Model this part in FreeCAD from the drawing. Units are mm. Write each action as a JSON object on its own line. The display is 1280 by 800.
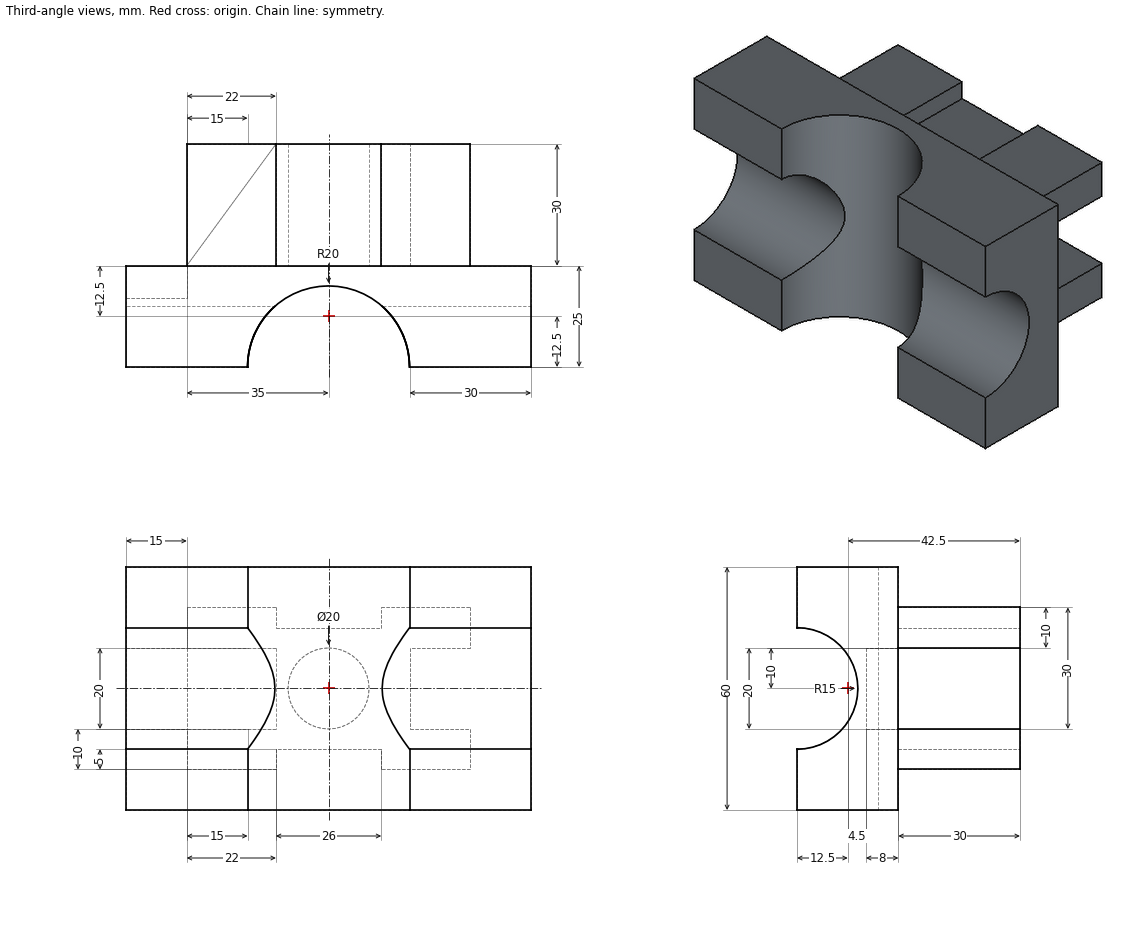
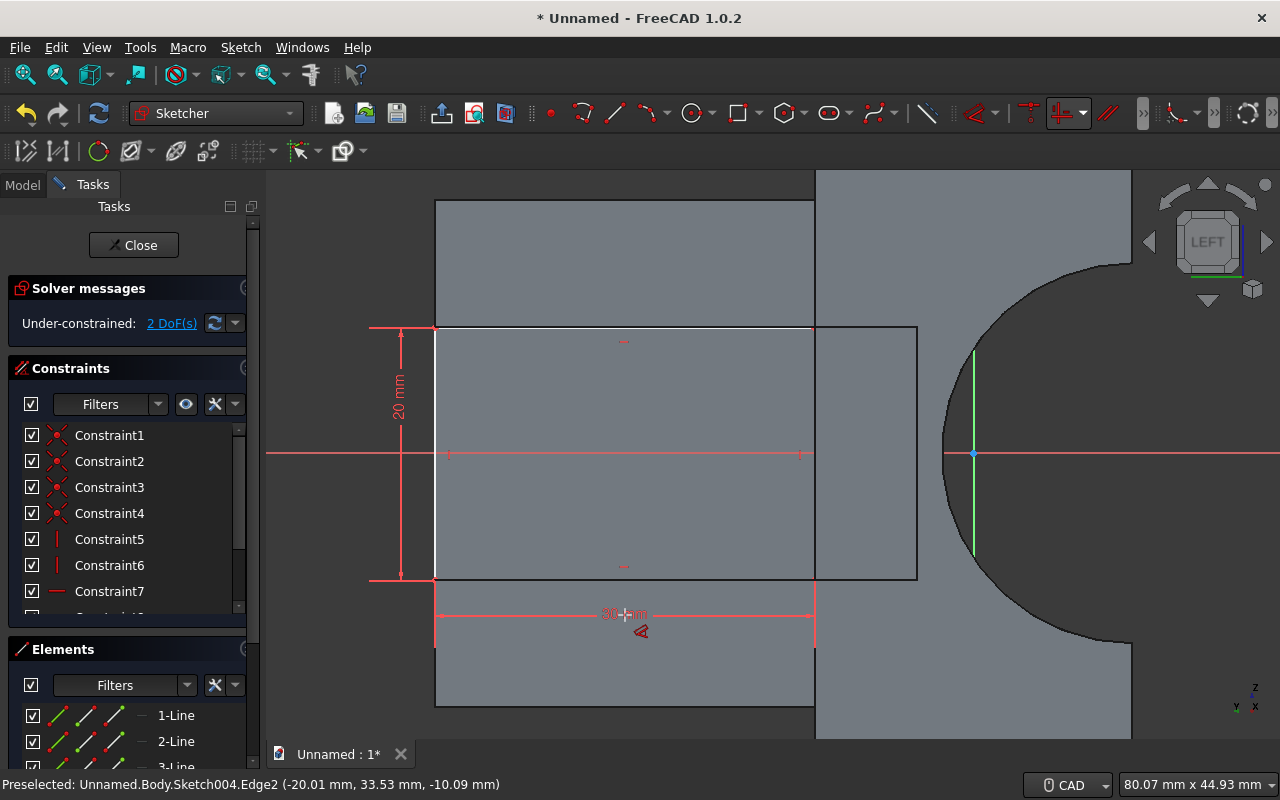
{"action": "left_click", "coordinate": [435, 328]}
{"action": "left_click", "coordinate": [401, 362]}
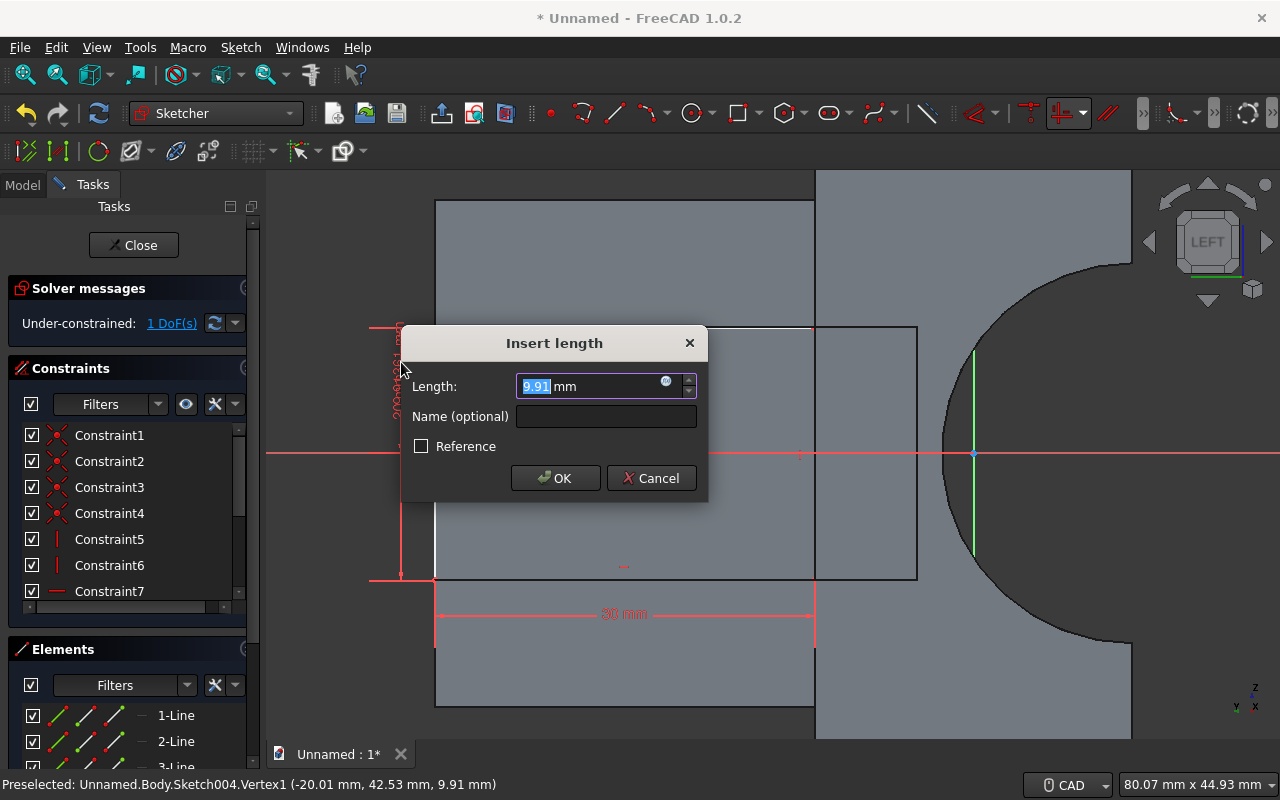
{"action": "type", "text": "10"}
{"action": "key", "text": "Return"}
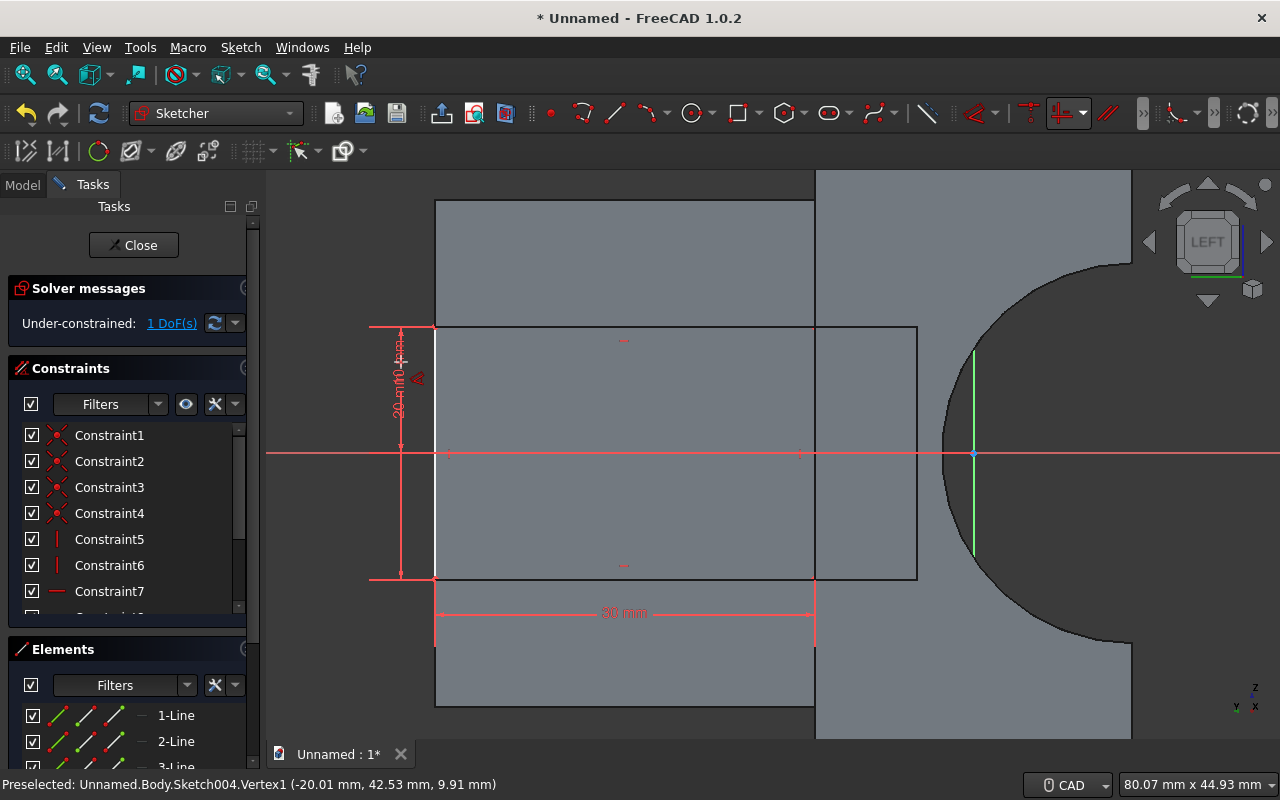
{"action": "left_click", "coordinate": [435, 327]}
{"action": "left_click", "coordinate": [704, 293]}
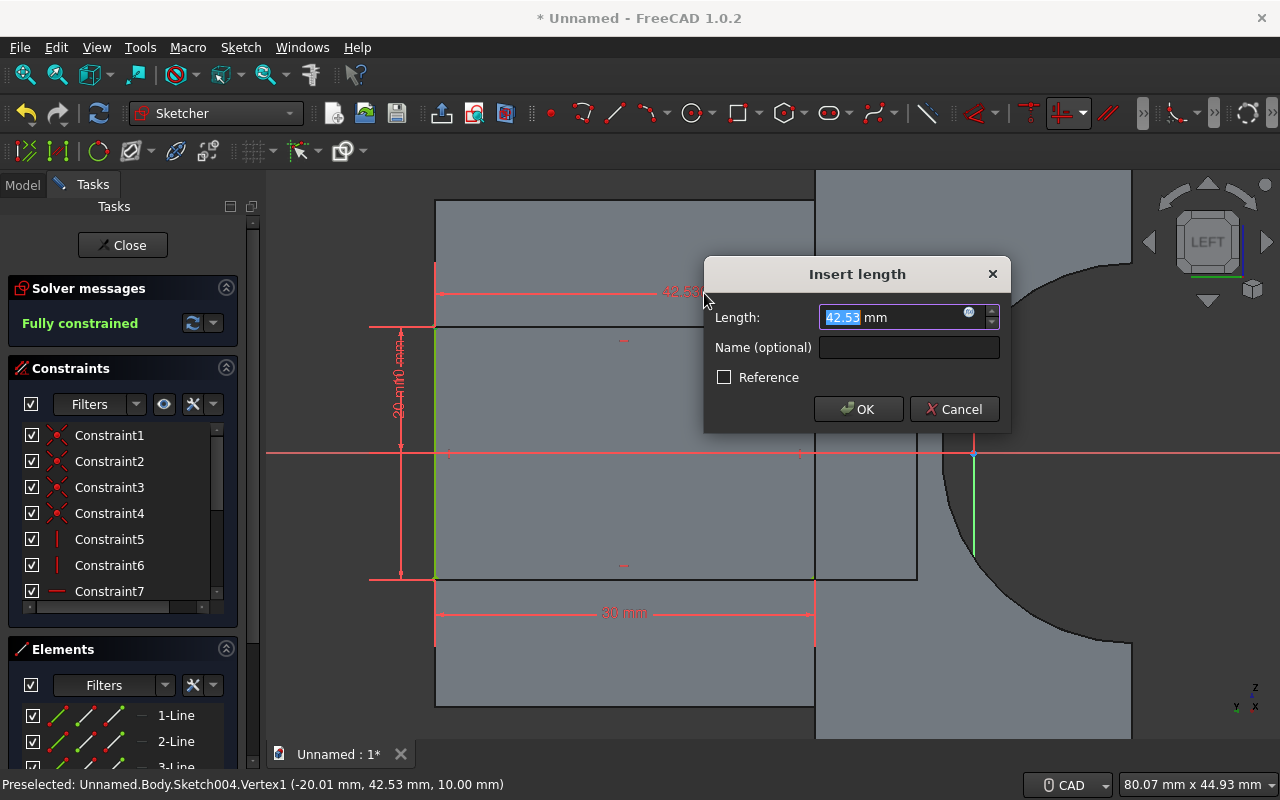
{"action": "type", "text": "42.5"}
{"action": "key", "text": "Return"}
{"action": "key", "text": "Escape"}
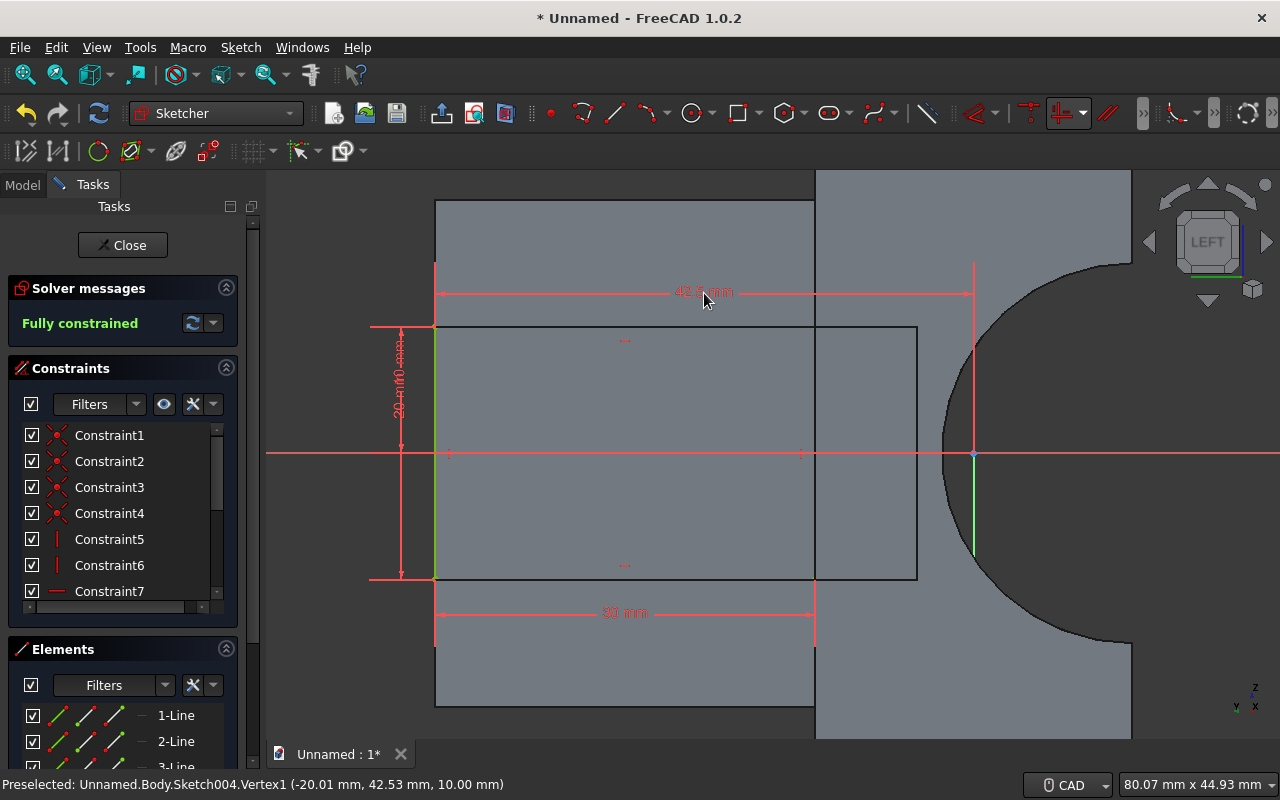
{"action": "left_click", "coordinate": [123, 245]}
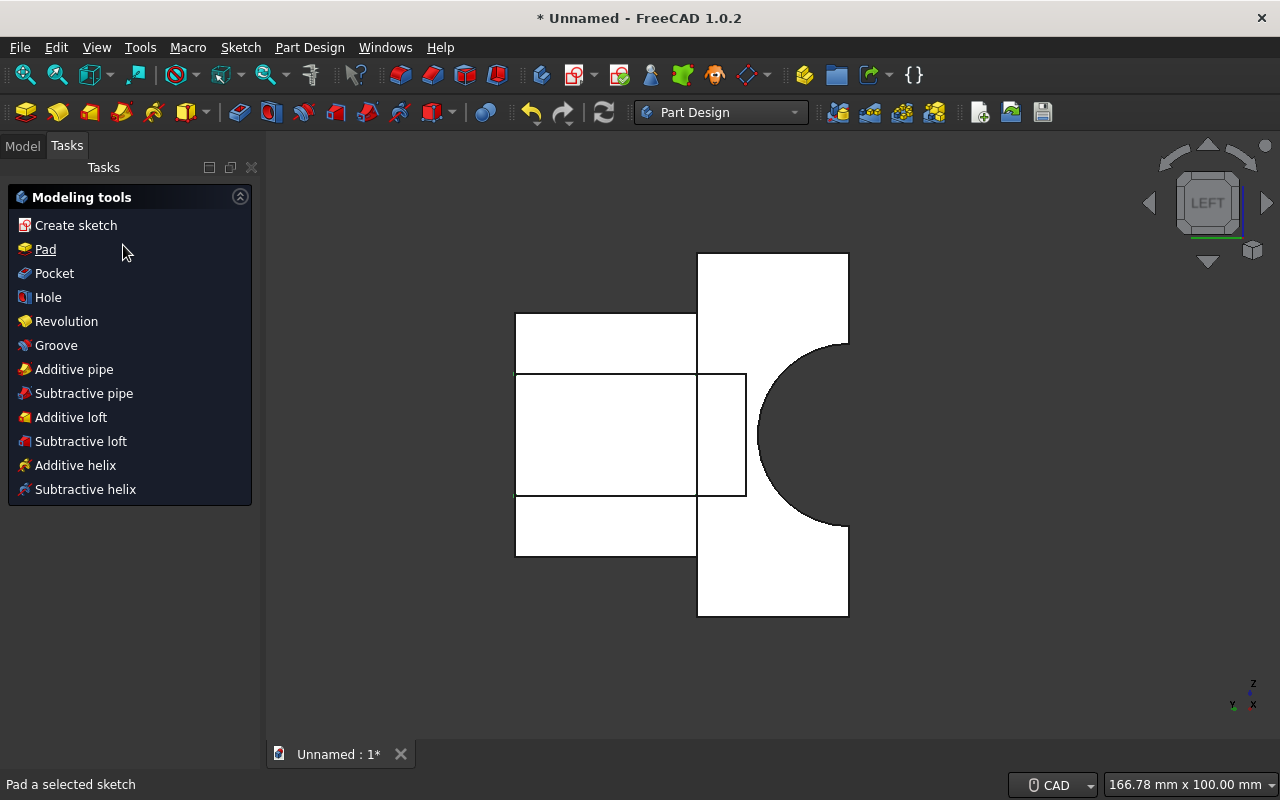
{"action": "left_click", "coordinate": [26, 112]}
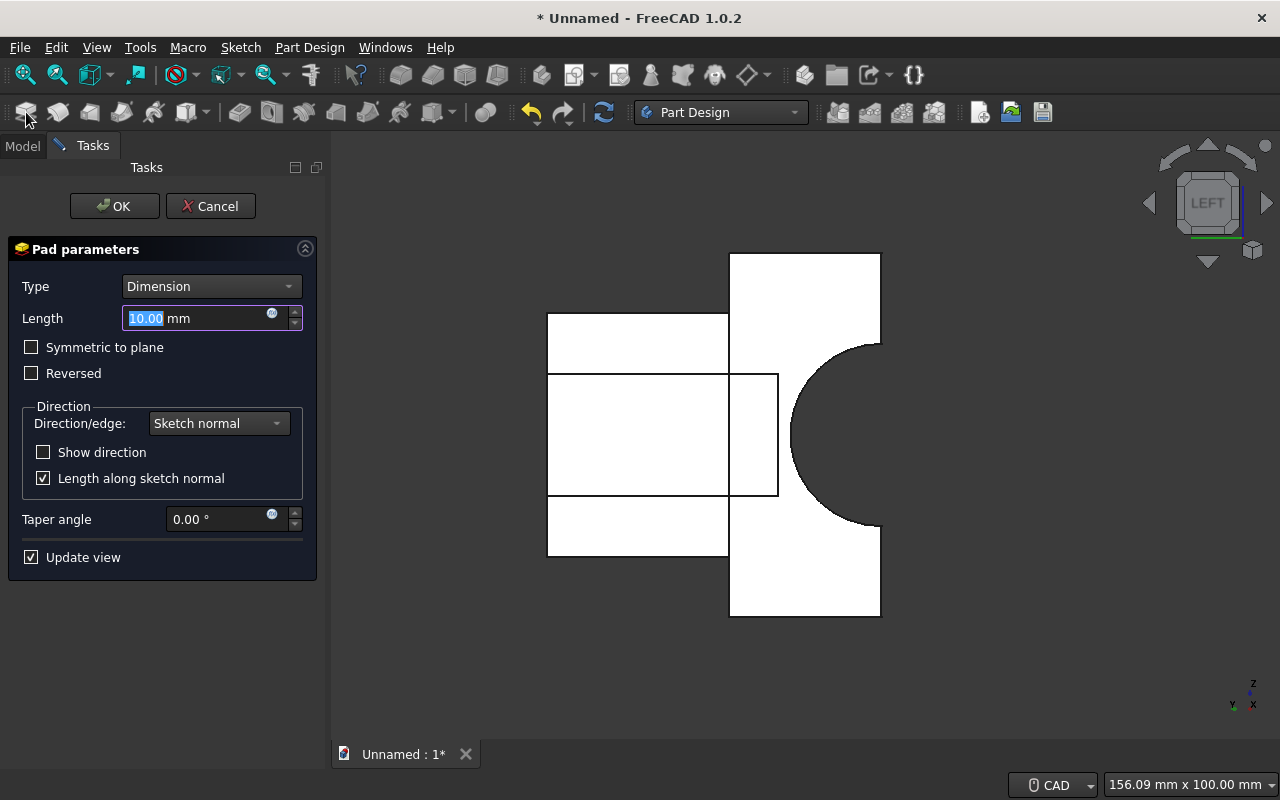
{"action": "type", "text": "15"}
{"action": "key", "text": "Tab"}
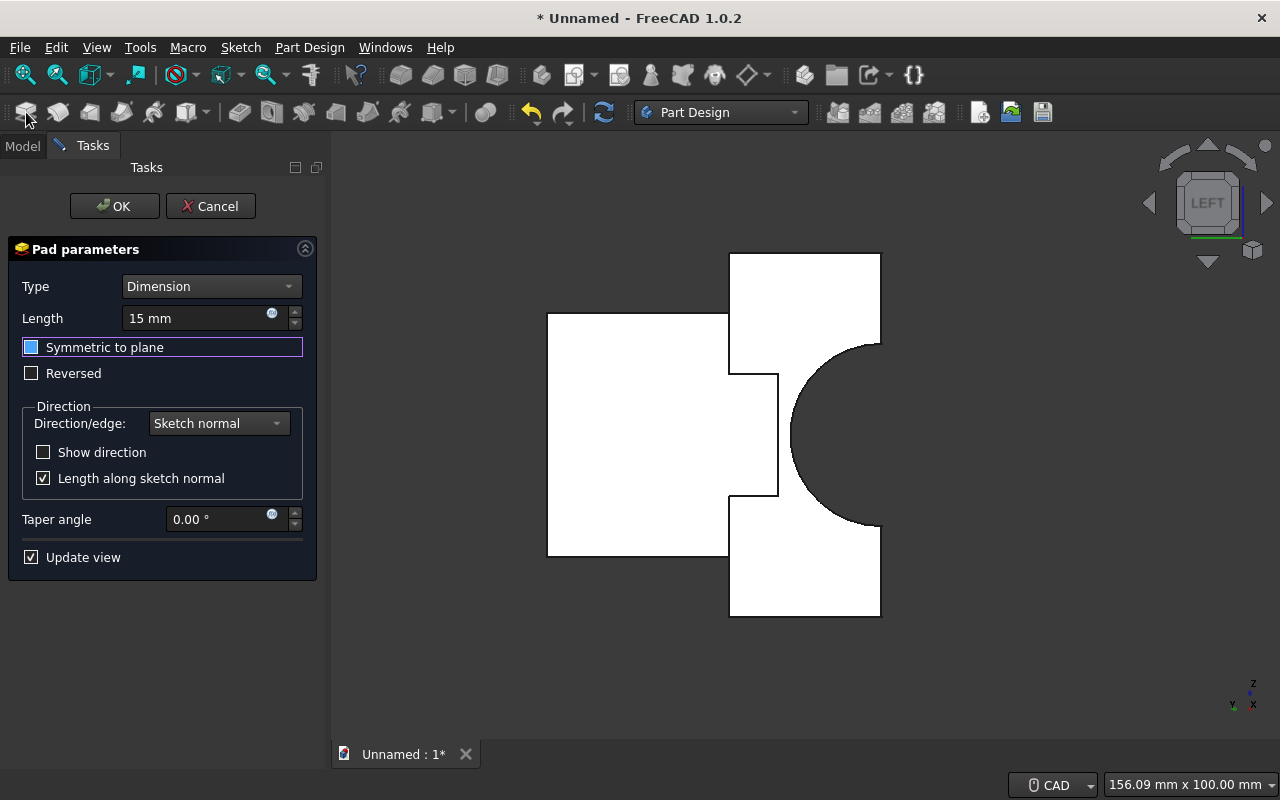
{"action": "left_click", "coordinate": [115, 206]}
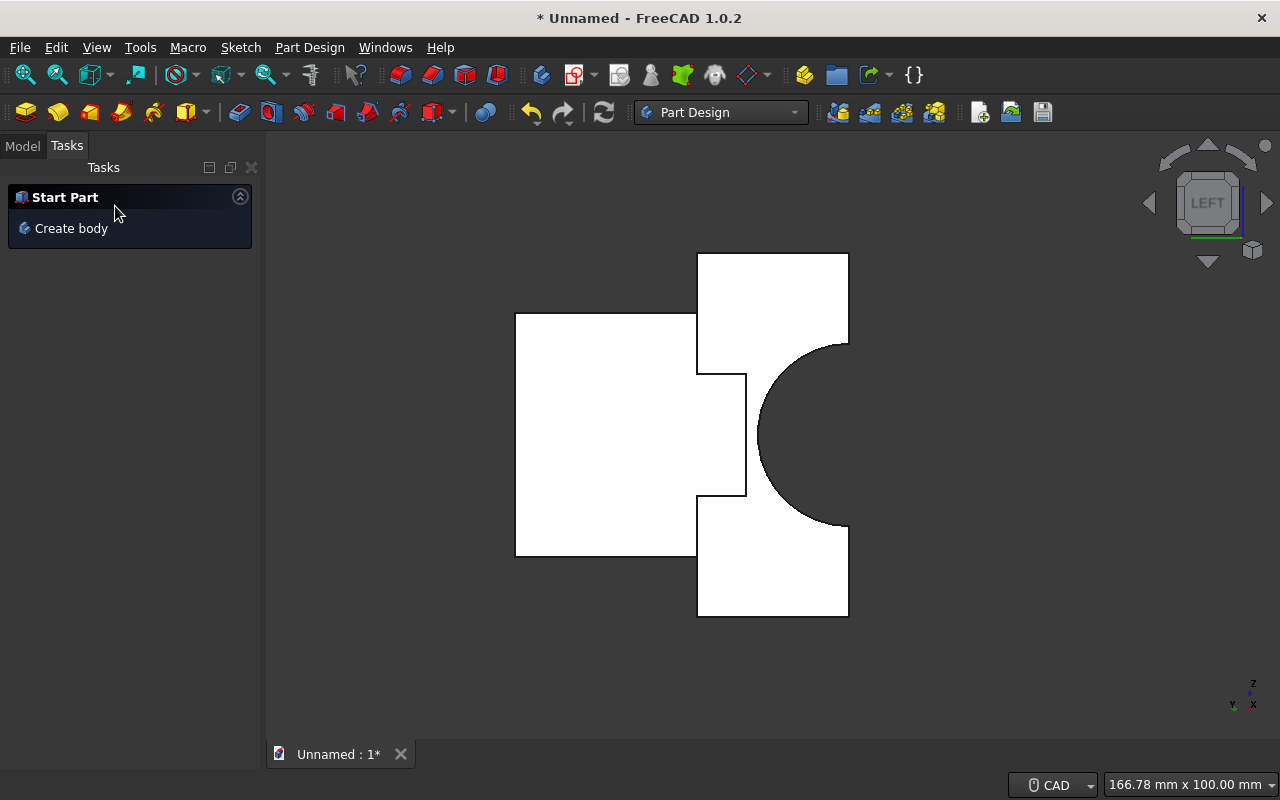
{"action": "key", "text": "0"}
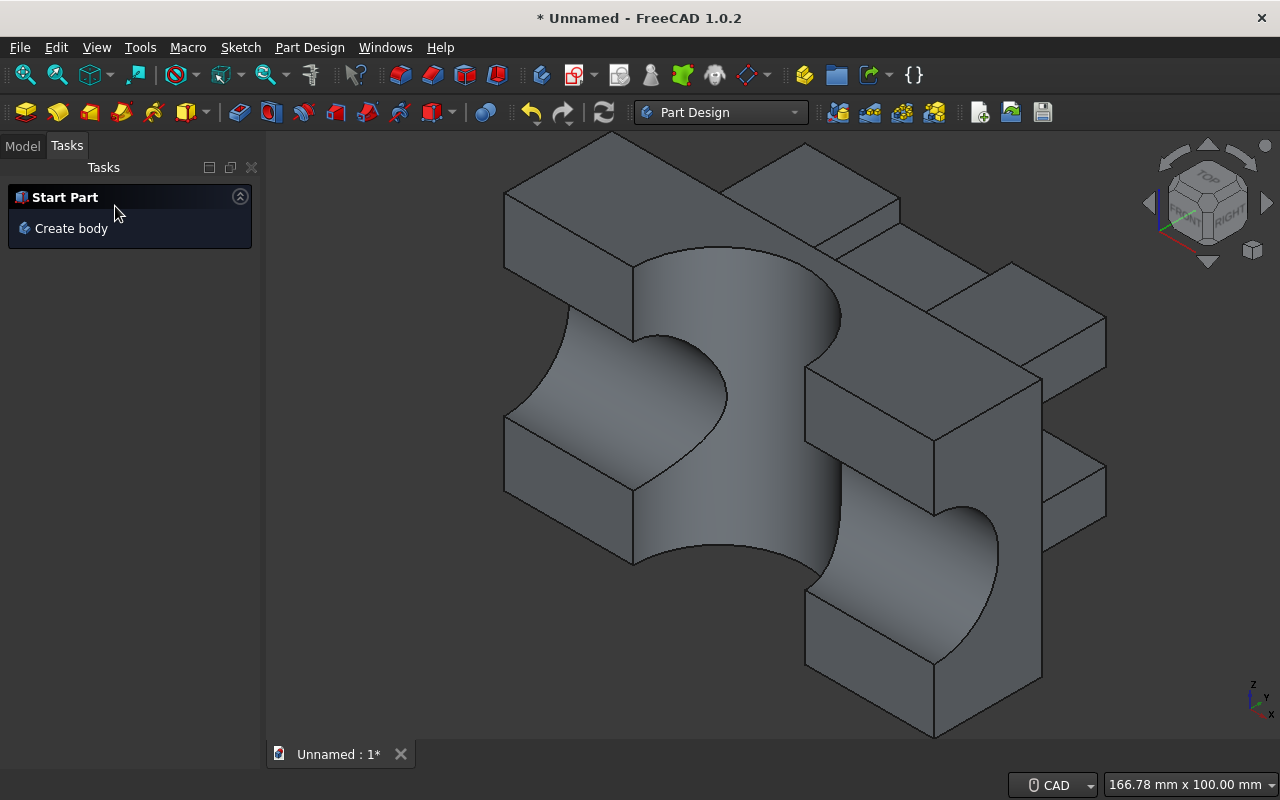
{"action": "left_click", "coordinate": [26, 76]}